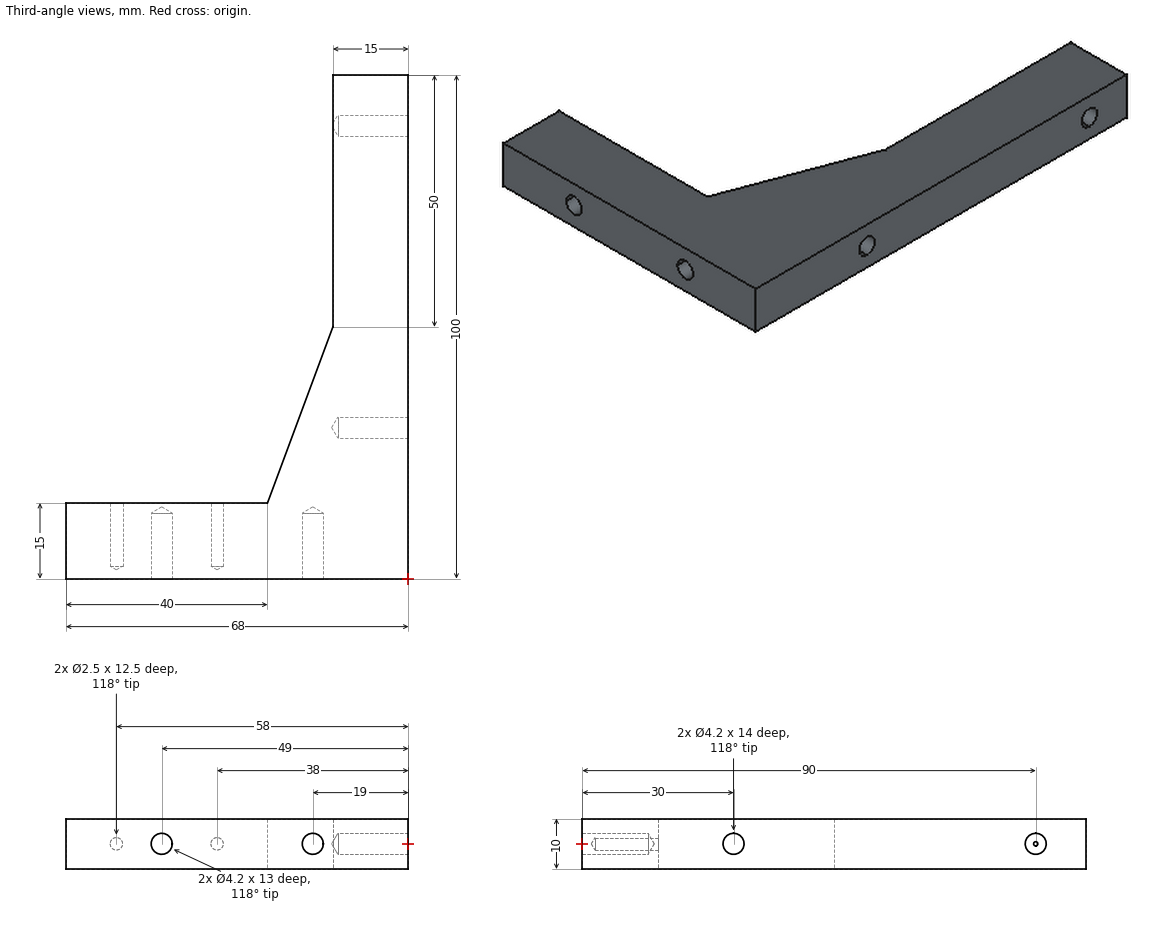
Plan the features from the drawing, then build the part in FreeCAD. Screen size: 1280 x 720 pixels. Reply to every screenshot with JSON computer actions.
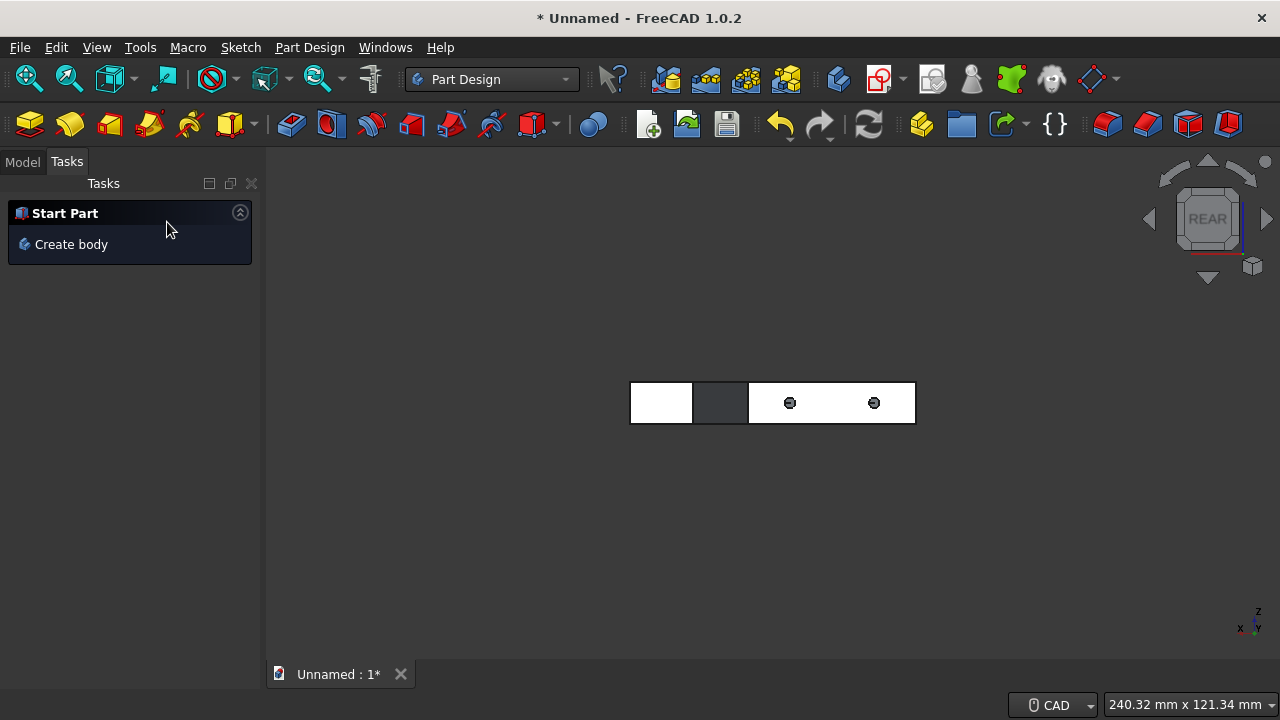
{"action": "key", "text": "0"}